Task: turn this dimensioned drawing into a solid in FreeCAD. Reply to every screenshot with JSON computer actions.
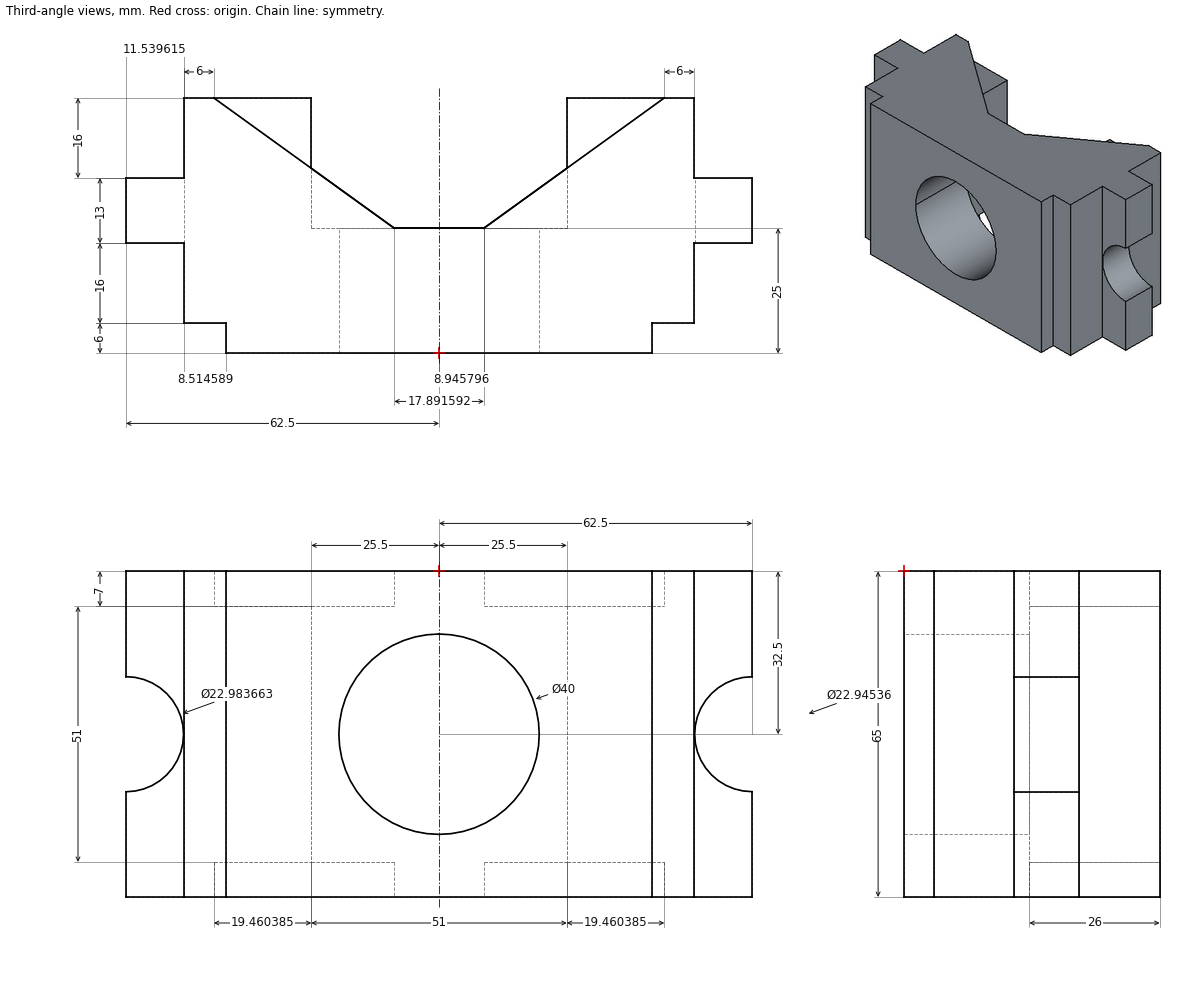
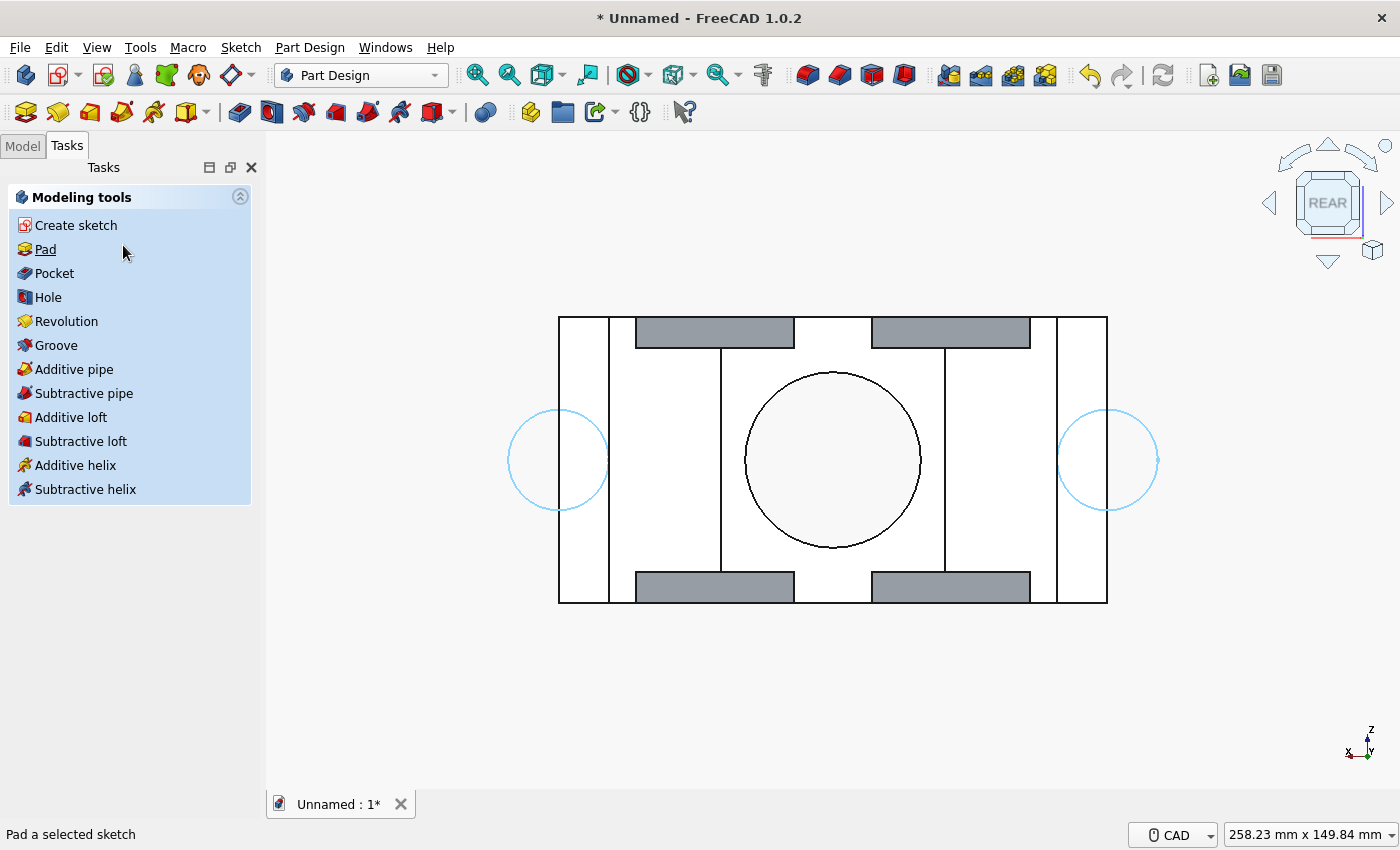
{"action": "left_click", "coordinate": [240, 112]}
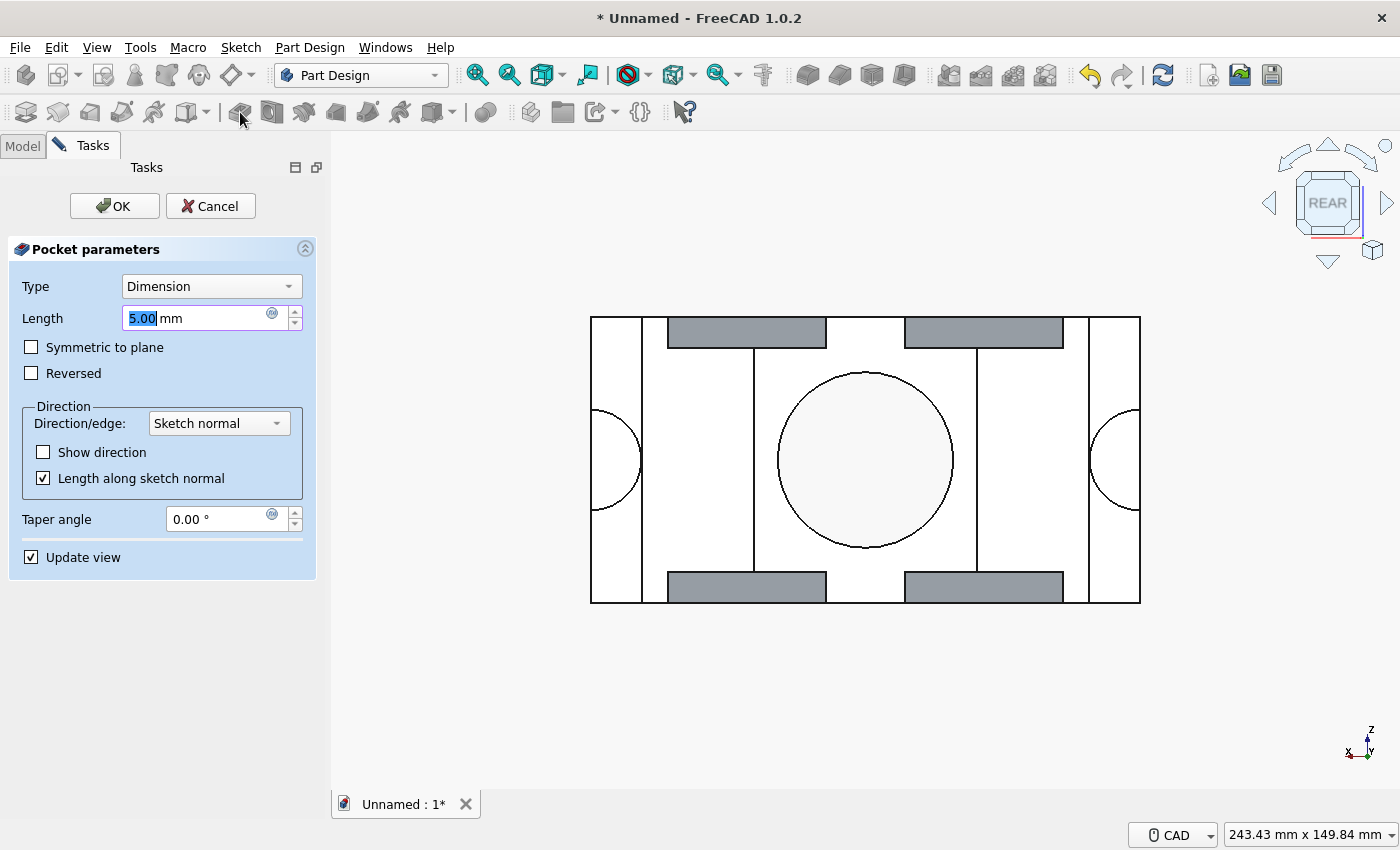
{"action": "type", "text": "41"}
{"action": "key", "text": "Tab"}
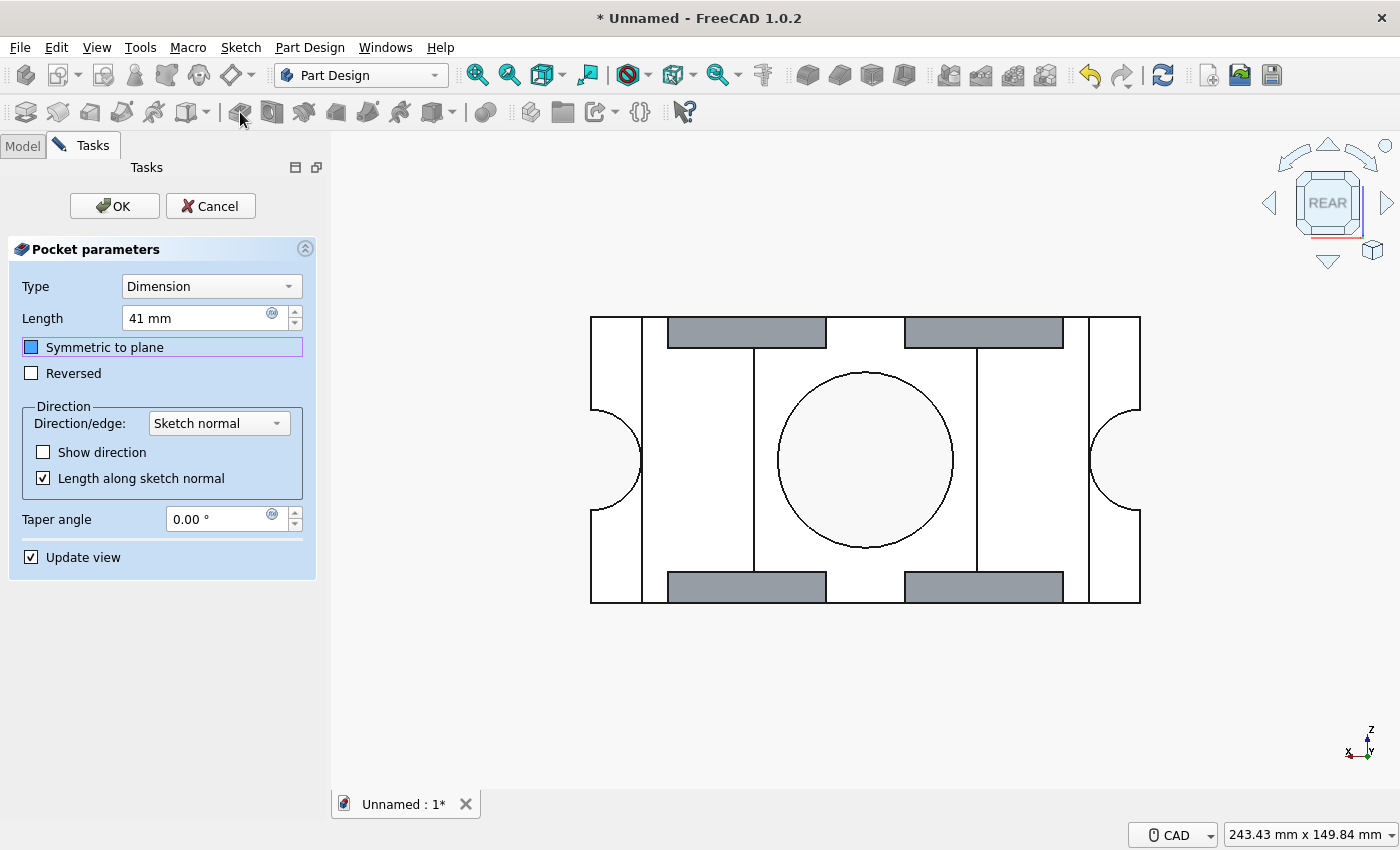
{"action": "left_click", "coordinate": [115, 206]}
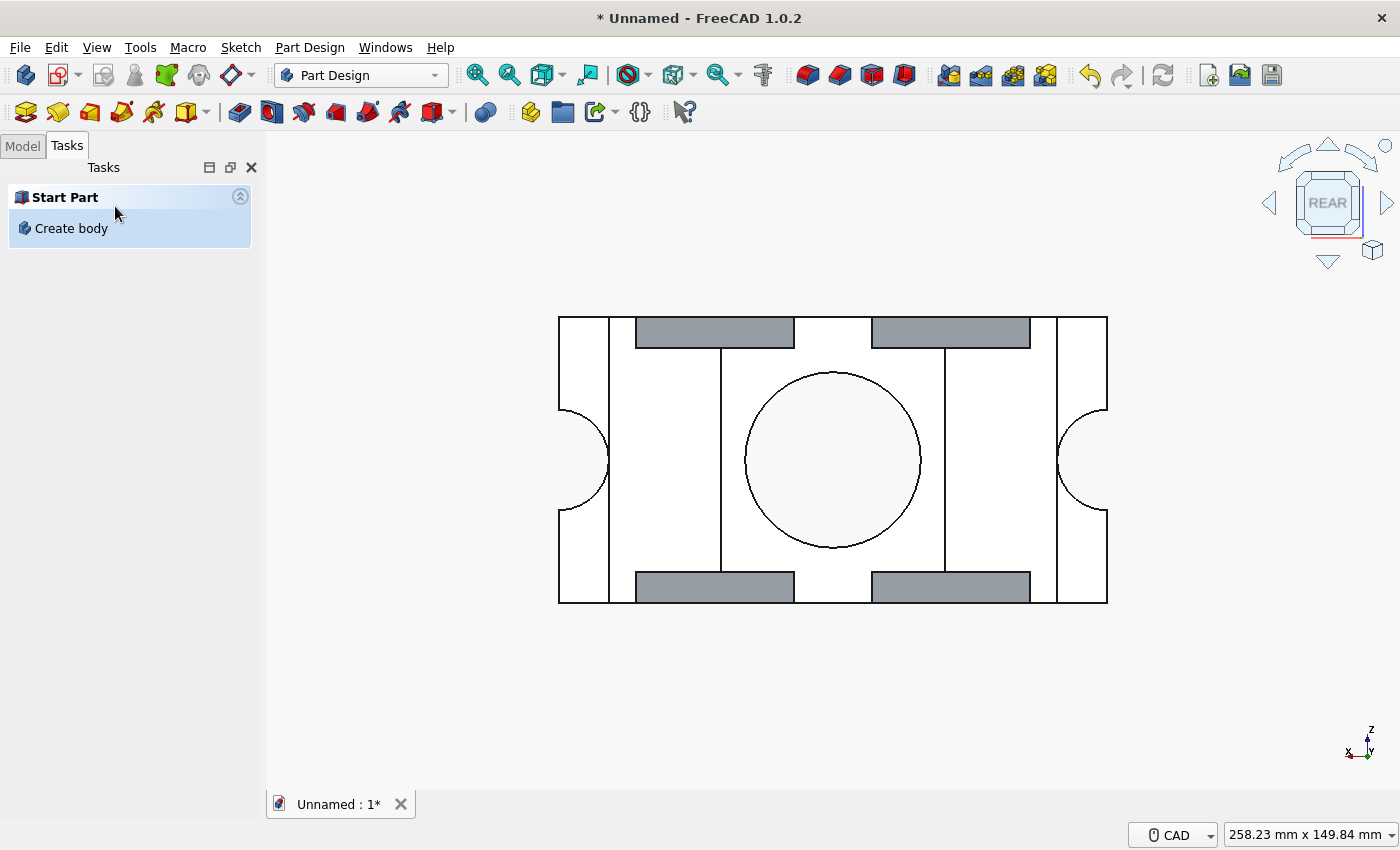
{"action": "key", "text": "0"}